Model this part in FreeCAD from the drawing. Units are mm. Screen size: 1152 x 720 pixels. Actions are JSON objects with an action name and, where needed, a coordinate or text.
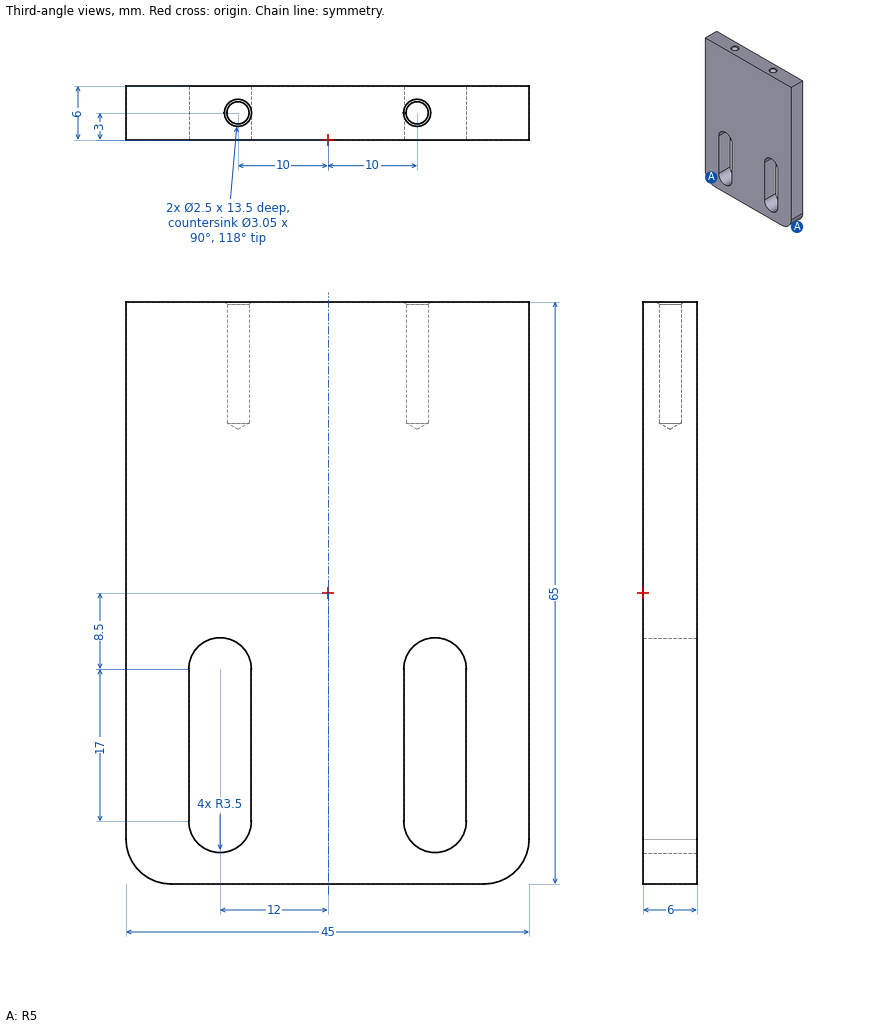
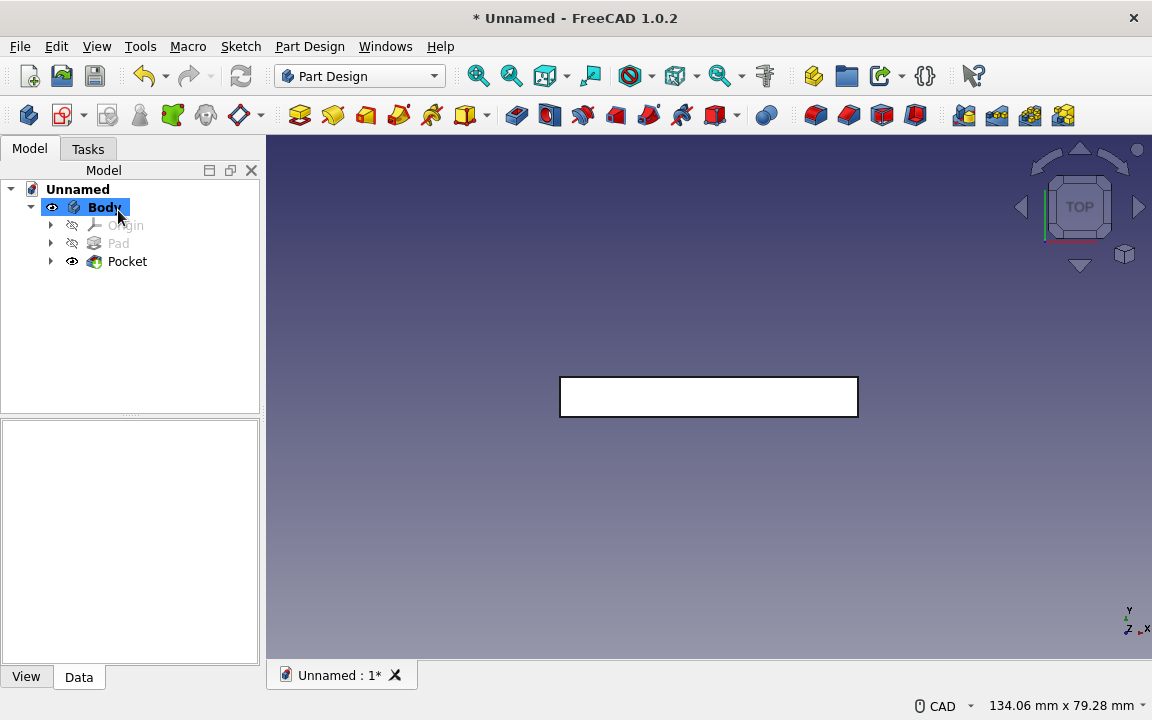
{"action": "key", "text": "1"}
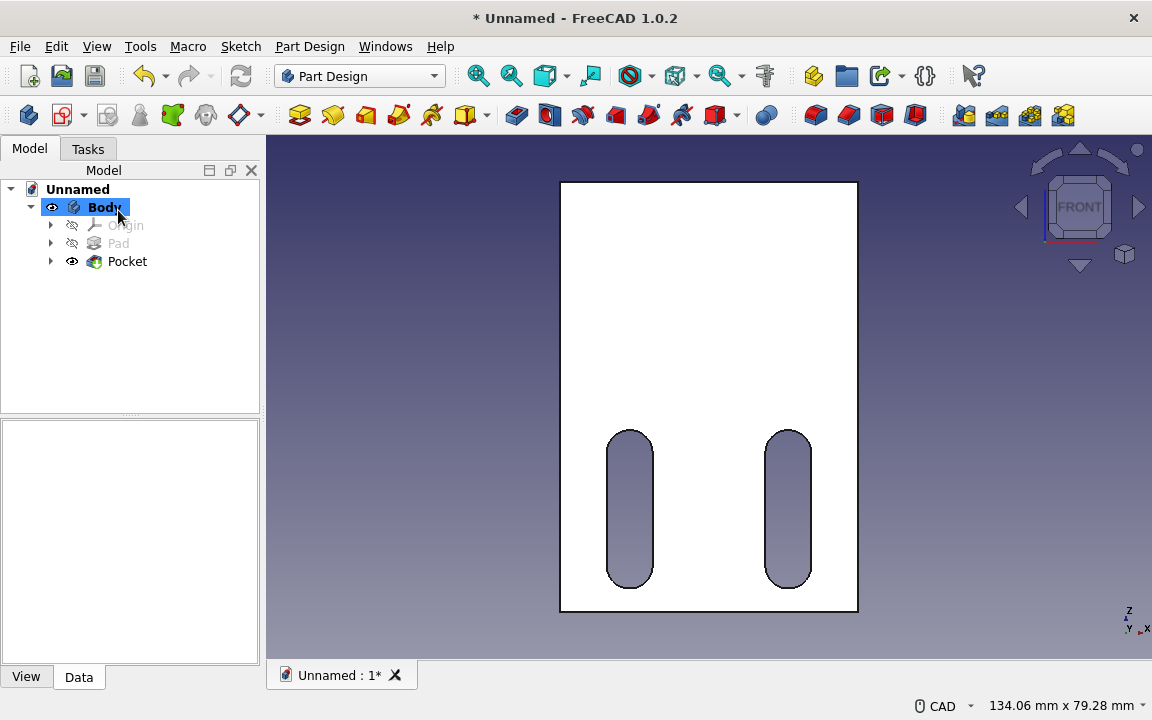
{"action": "key", "text": "3"}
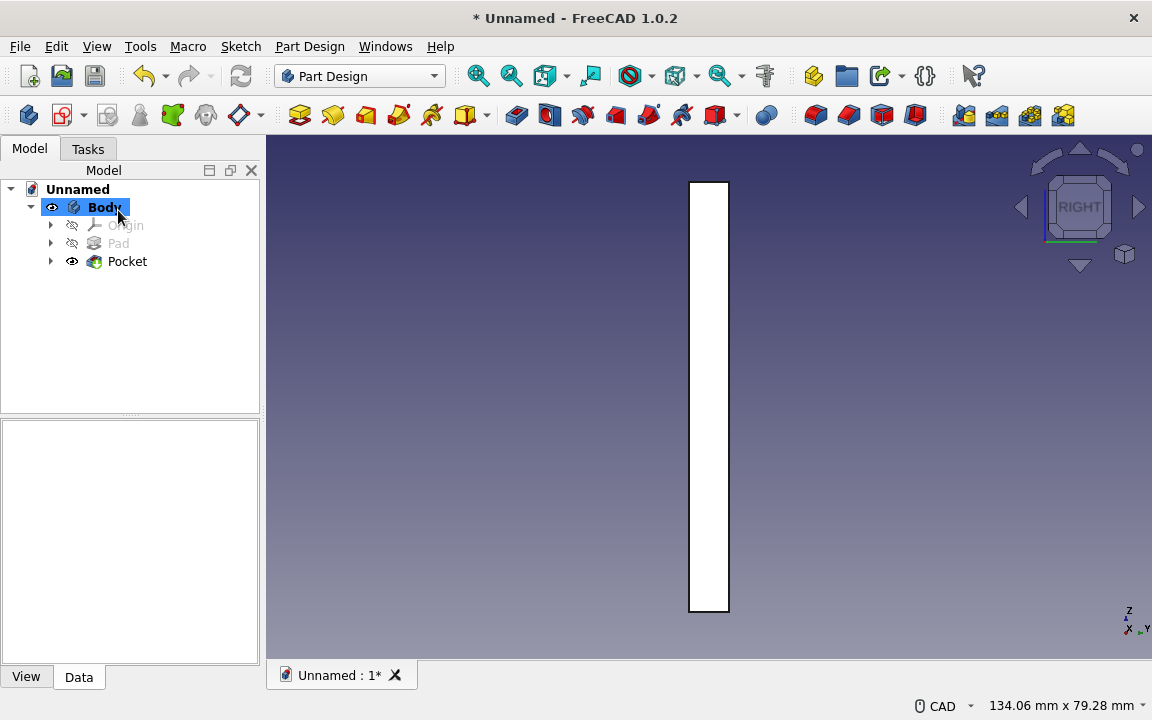
{"action": "left_click", "coordinate": [709, 611]}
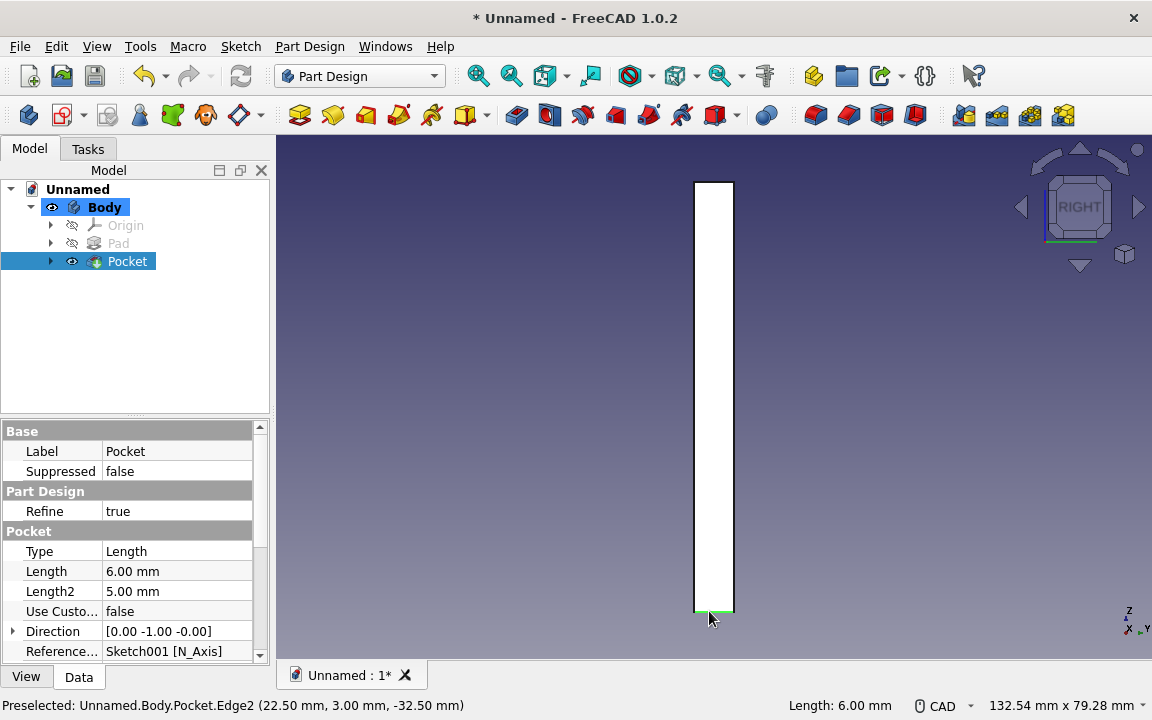
{"action": "key", "text": "5"}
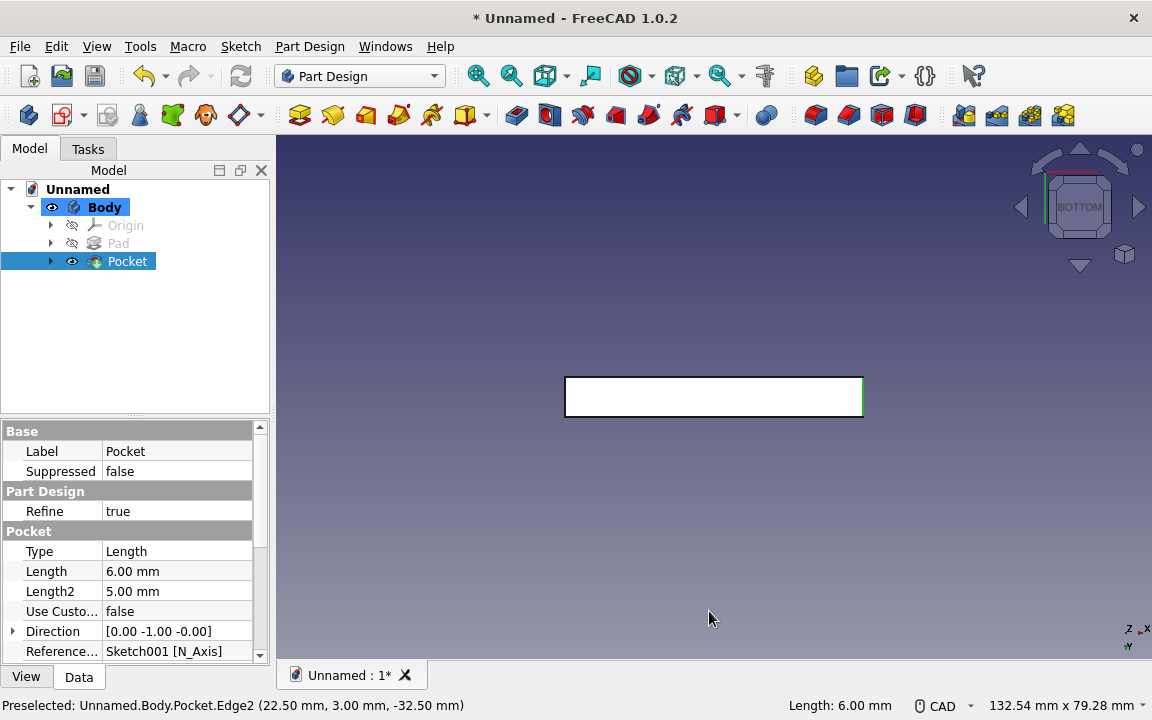
{"action": "key", "text": "v f"}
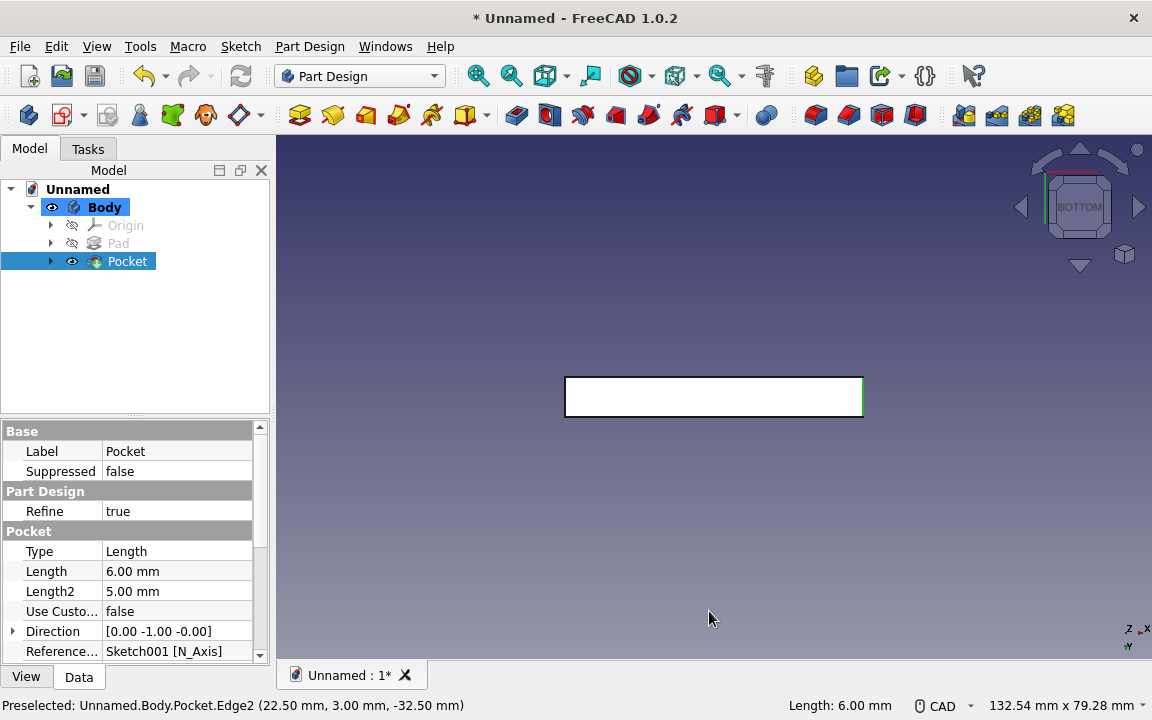
{"action": "left_click", "coordinate": [565, 396], "text": "ctrl"}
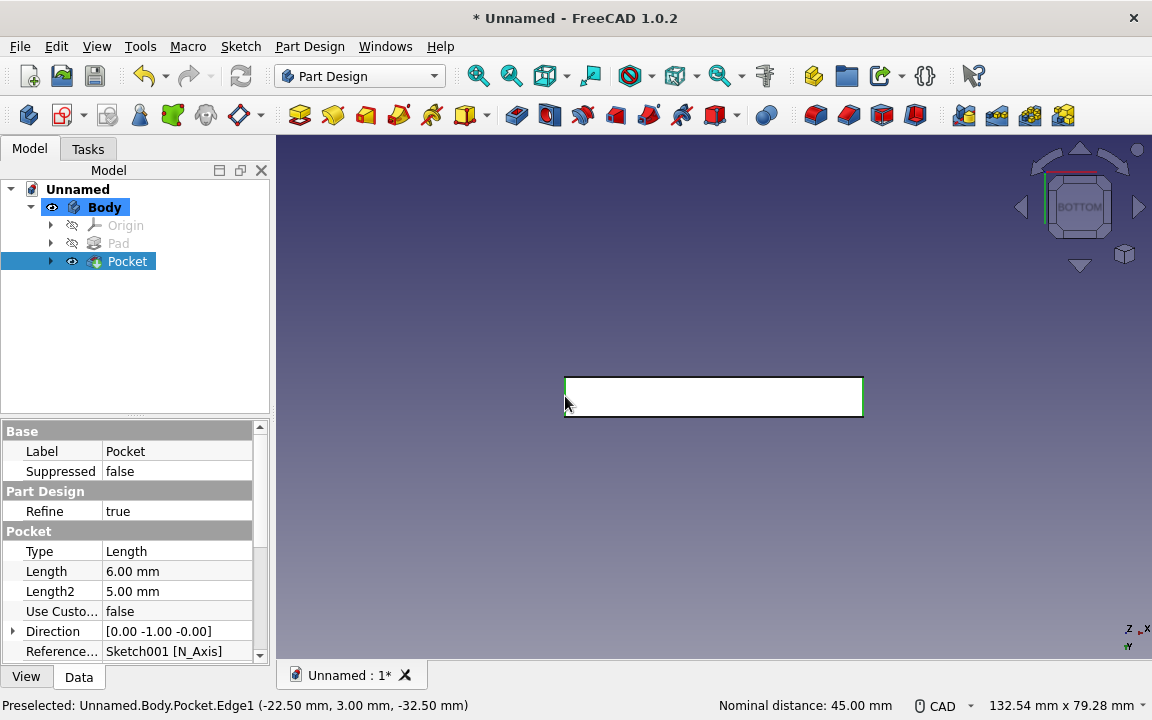
{"action": "left_click", "coordinate": [816, 116]}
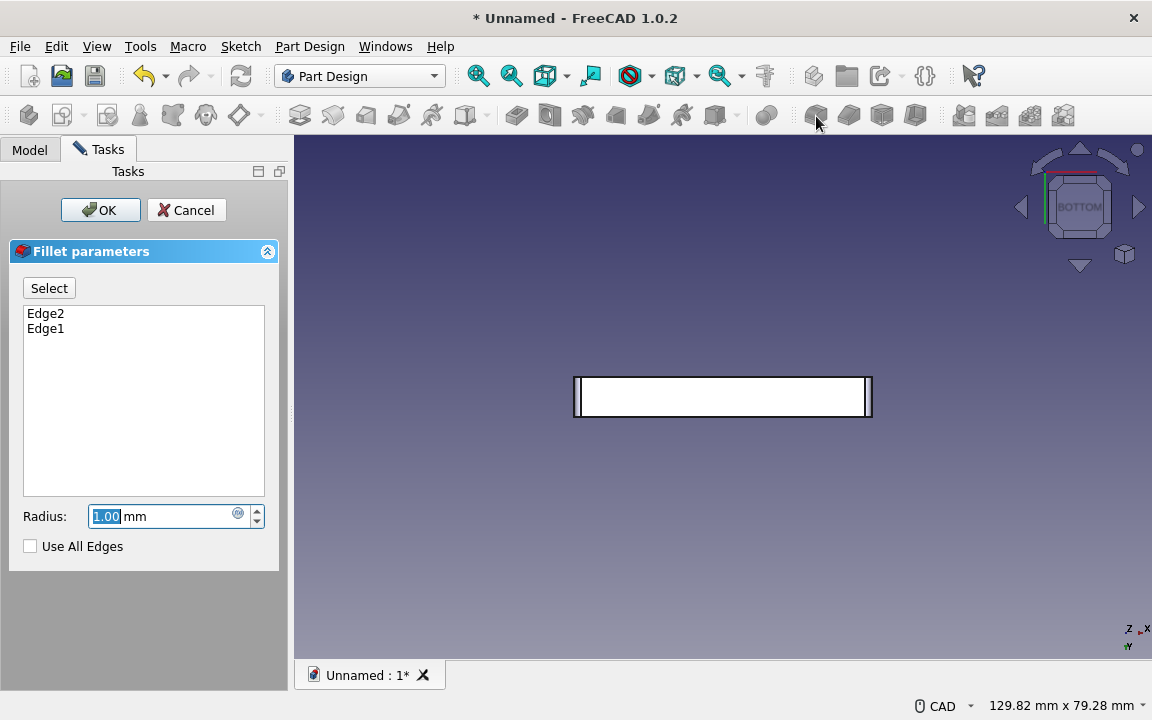
{"action": "type", "text": "5"}
{"action": "key", "text": "Tab"}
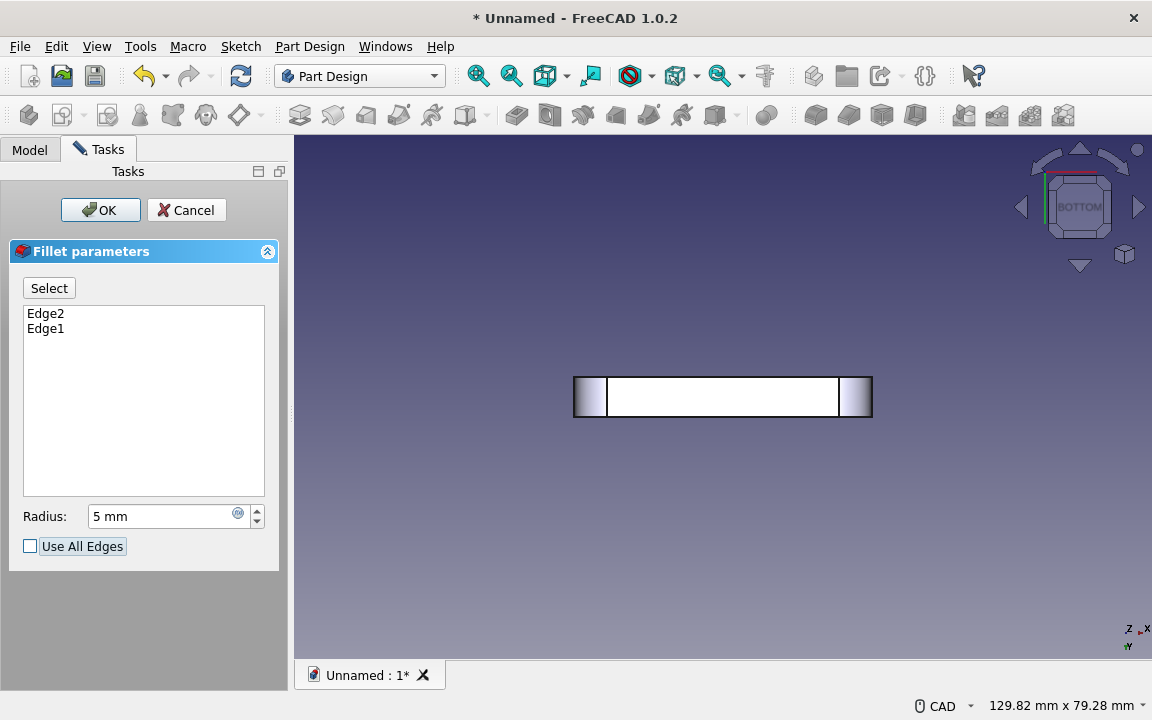
{"action": "left_click", "coordinate": [101, 210]}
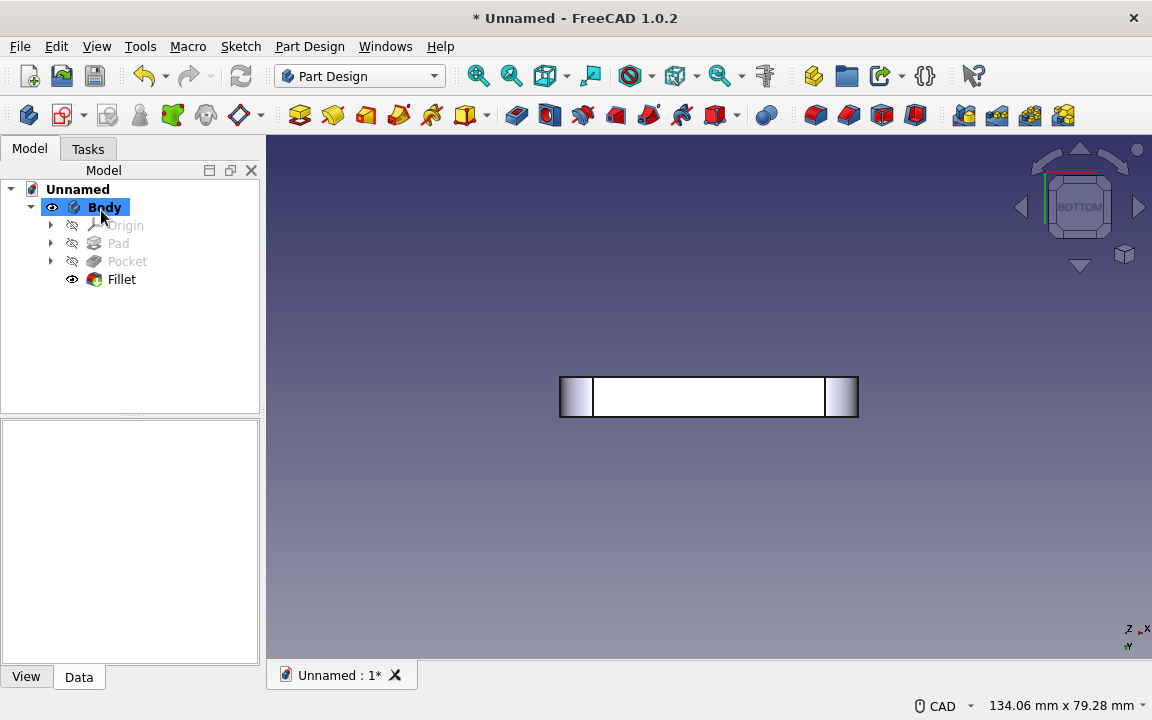
{"action": "left_click", "coordinate": [479, 76]}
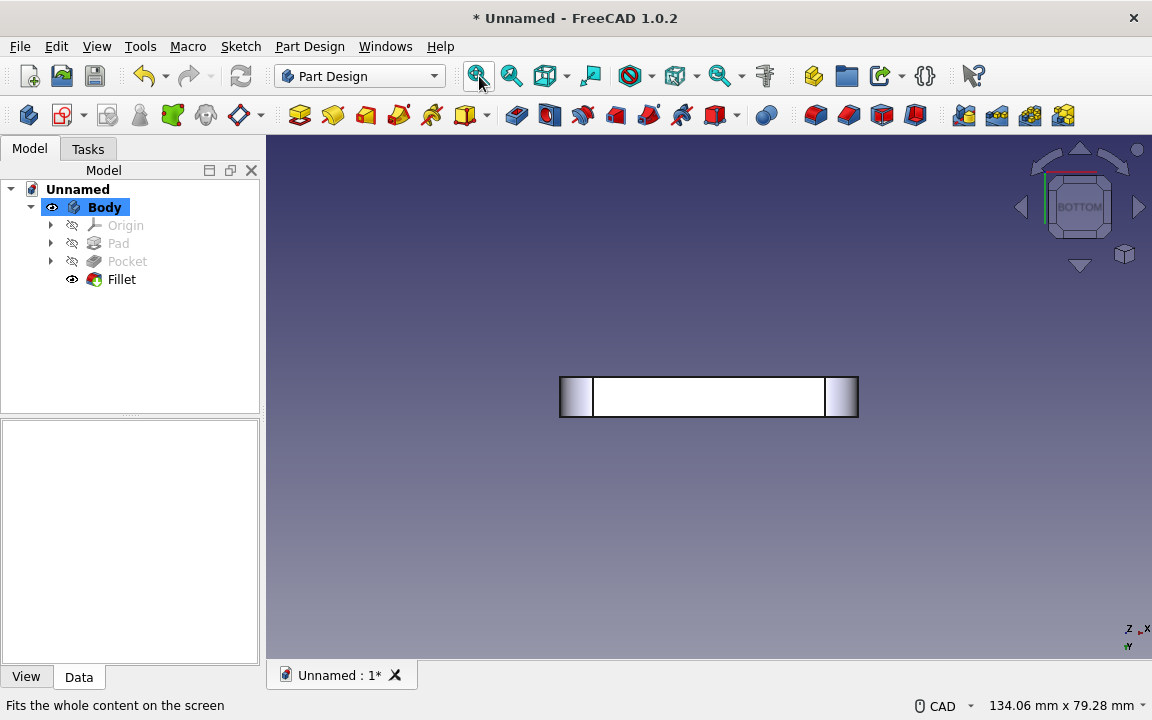
{"action": "key", "text": "0"}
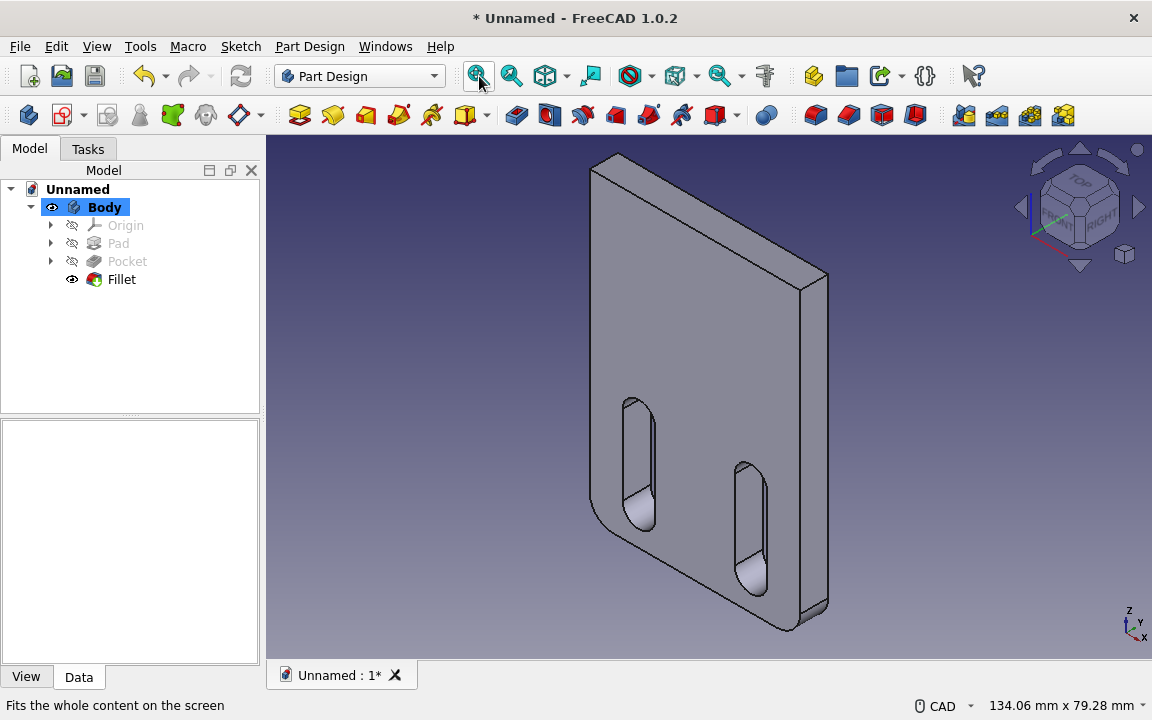
{"action": "left_click", "coordinate": [799, 273]}